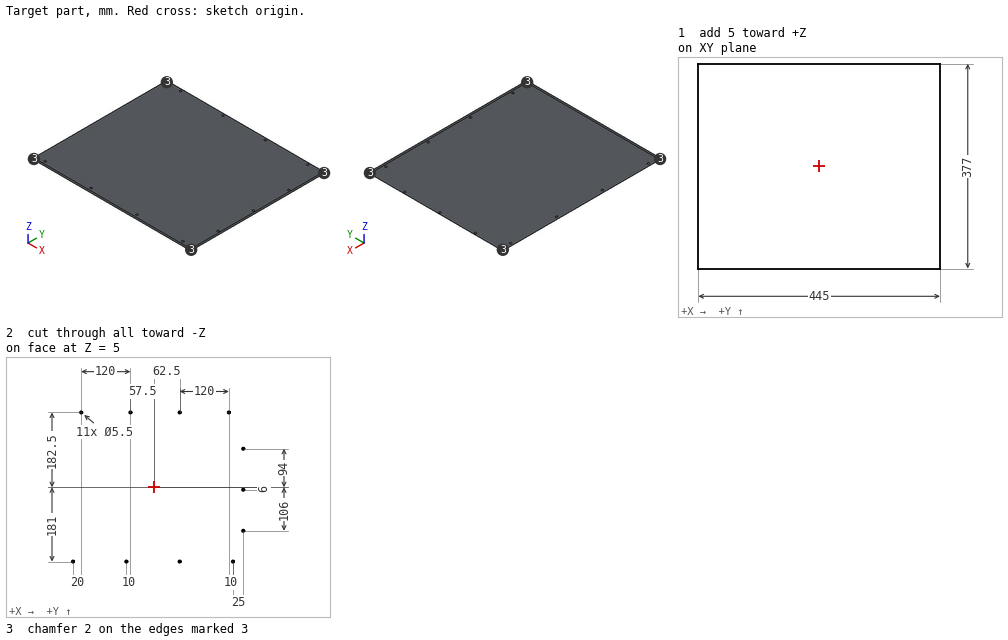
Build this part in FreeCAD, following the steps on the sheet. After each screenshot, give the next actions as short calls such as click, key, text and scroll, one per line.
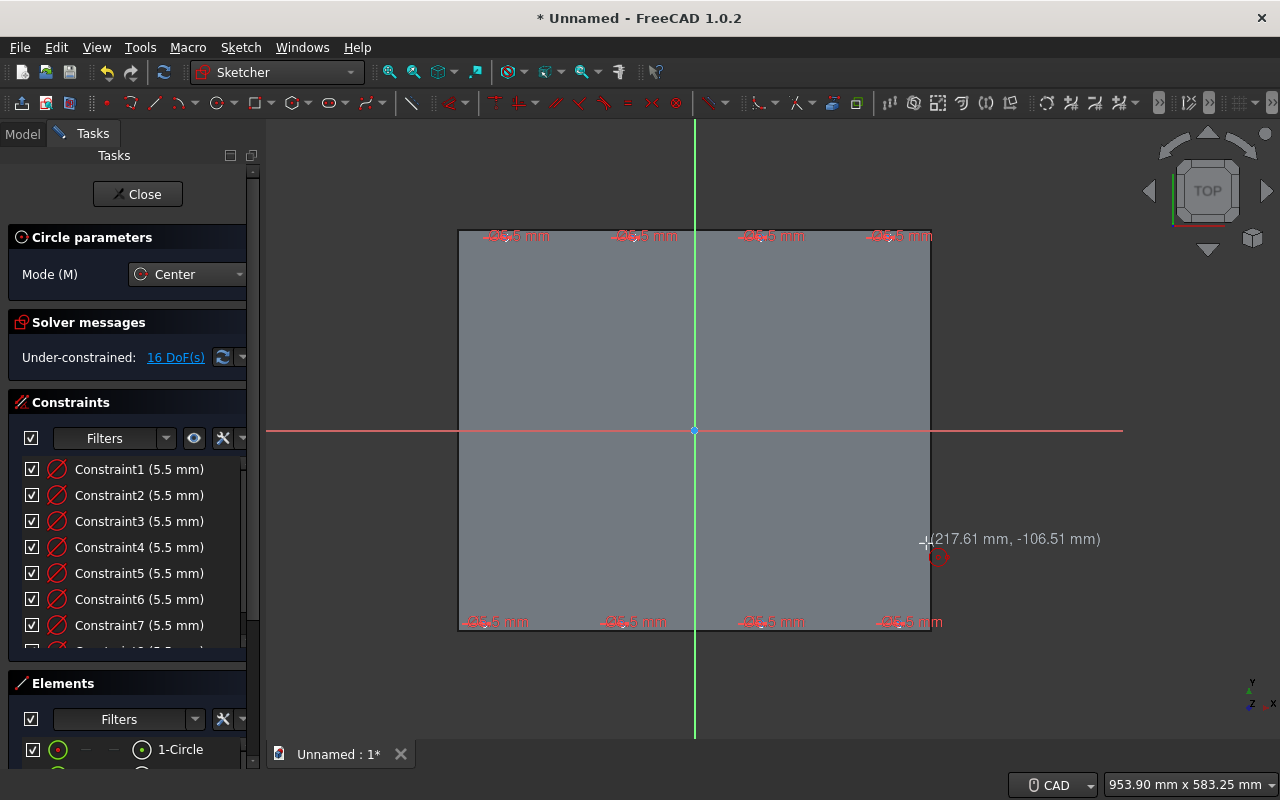
click(926, 543)
move(928, 541)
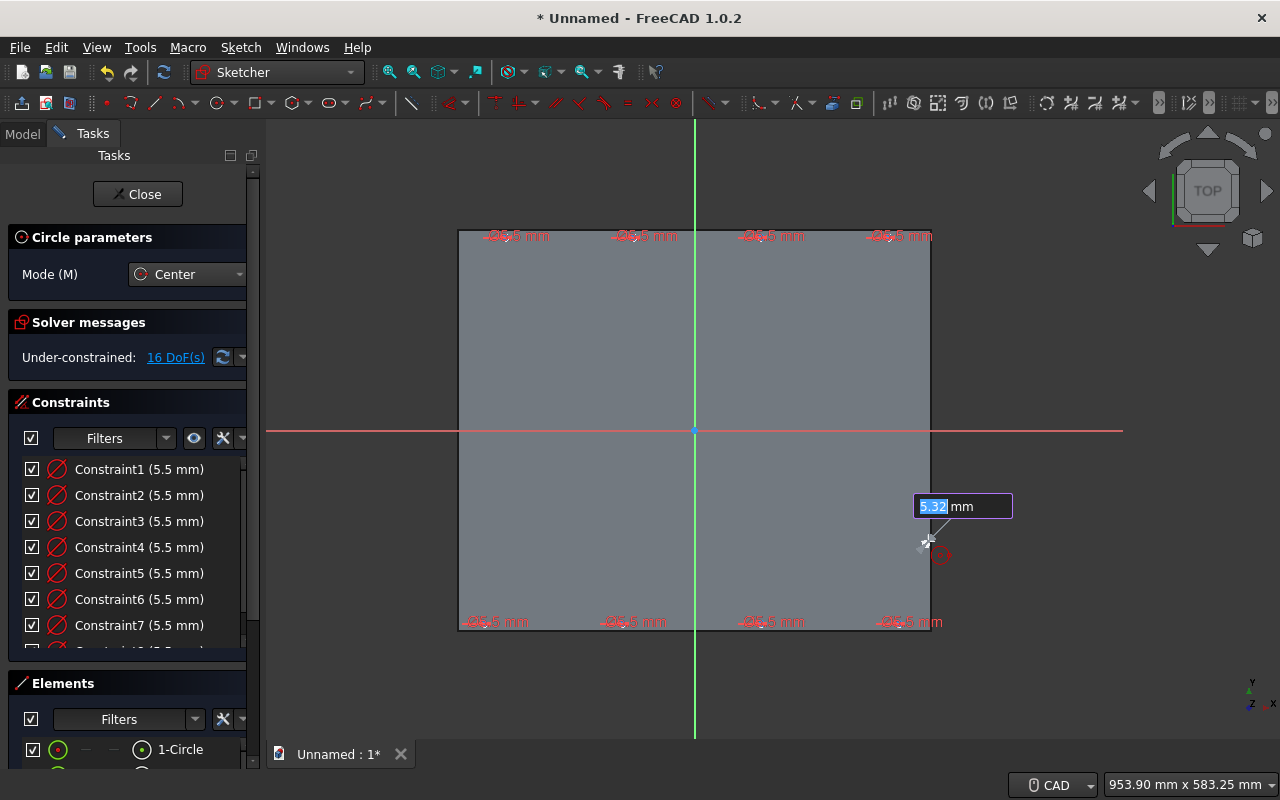
text(5.5)
key(Return)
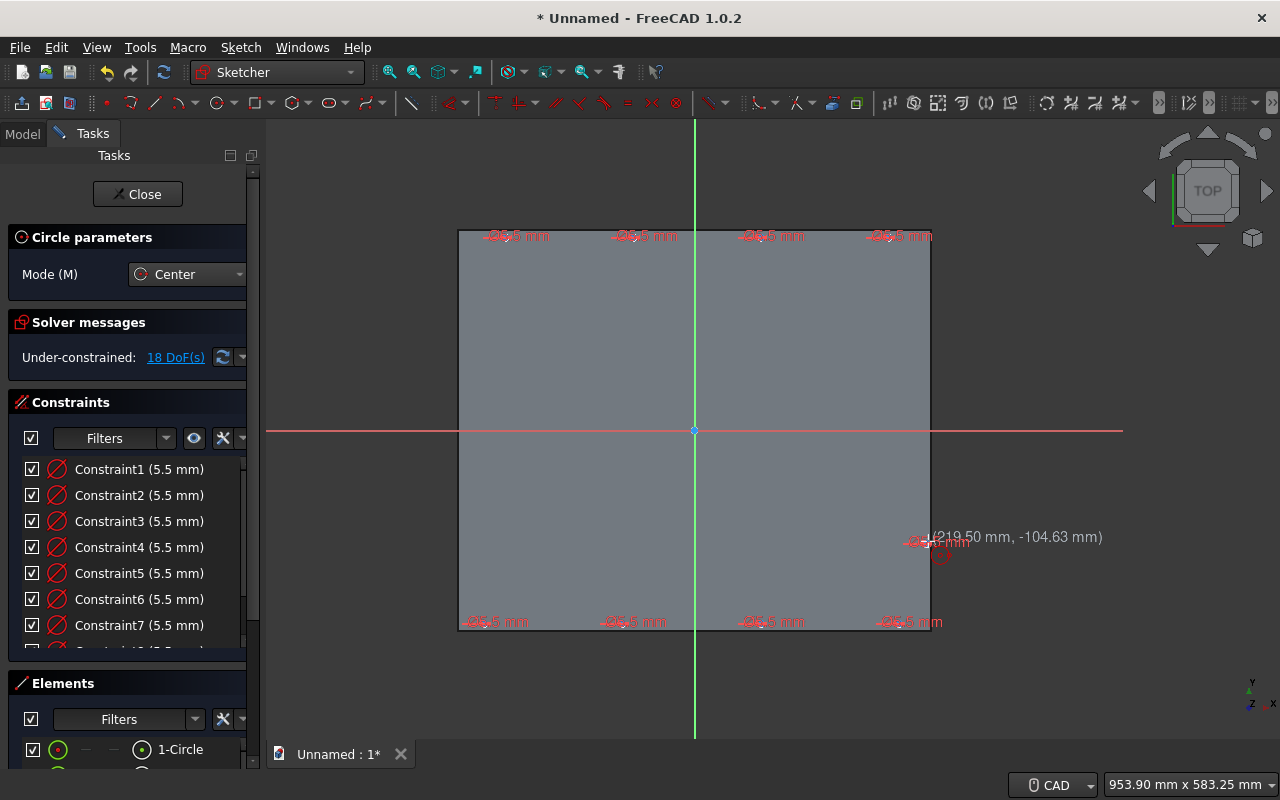
scroll(926, 437, up, 11)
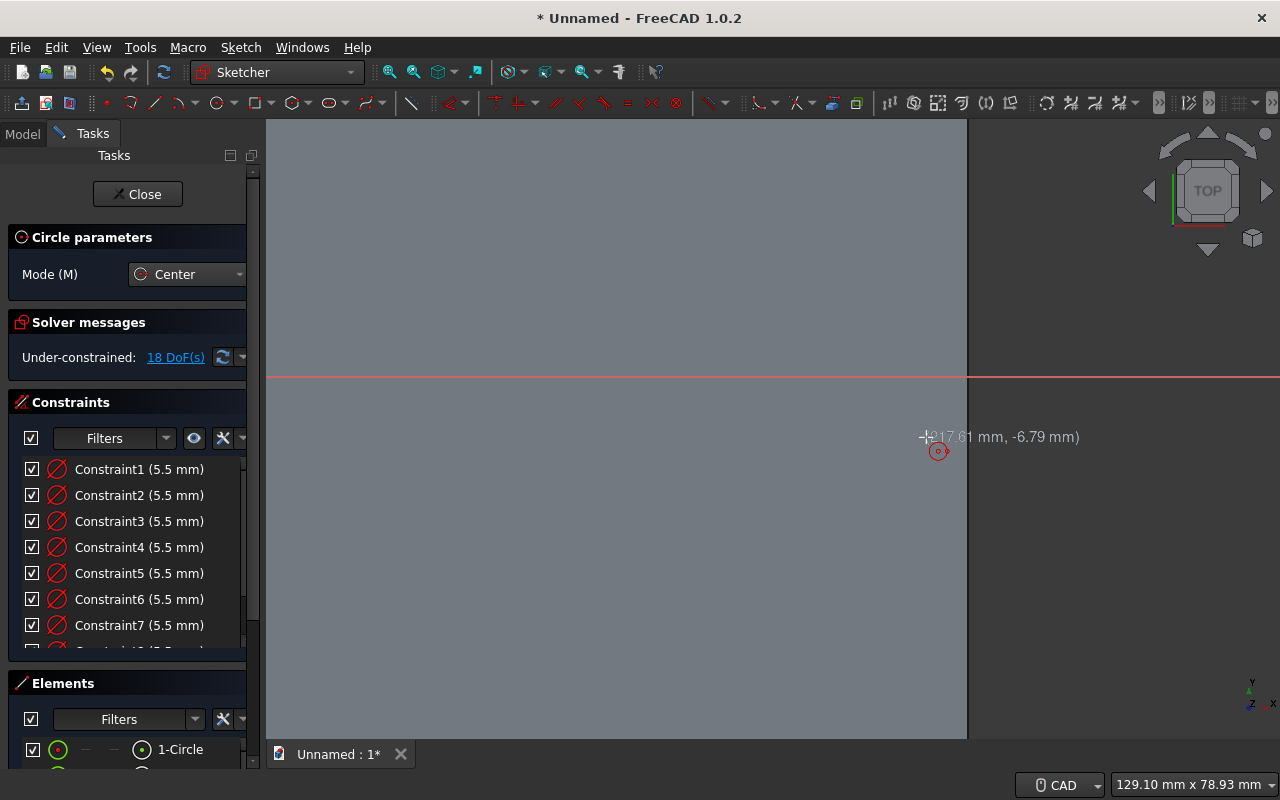
scroll(926, 436, down, 11)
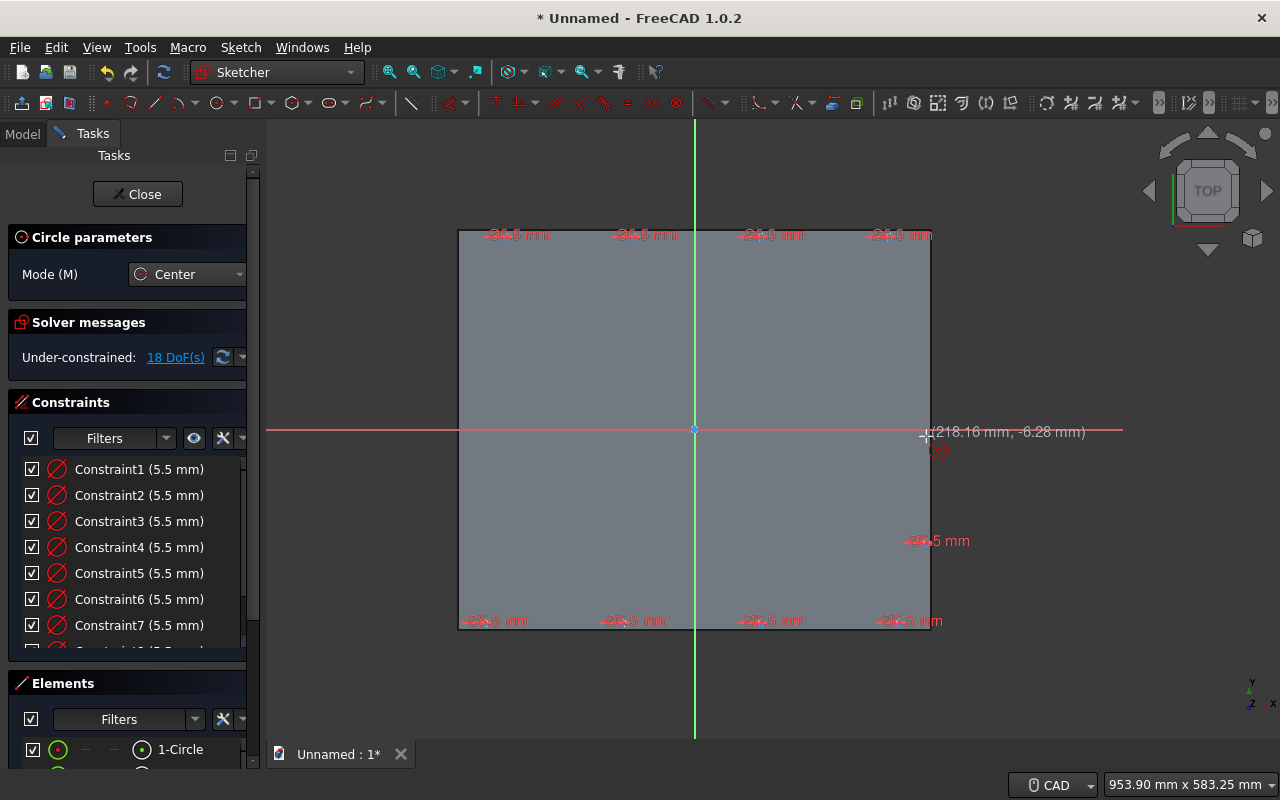
scroll(926, 436, up, 5)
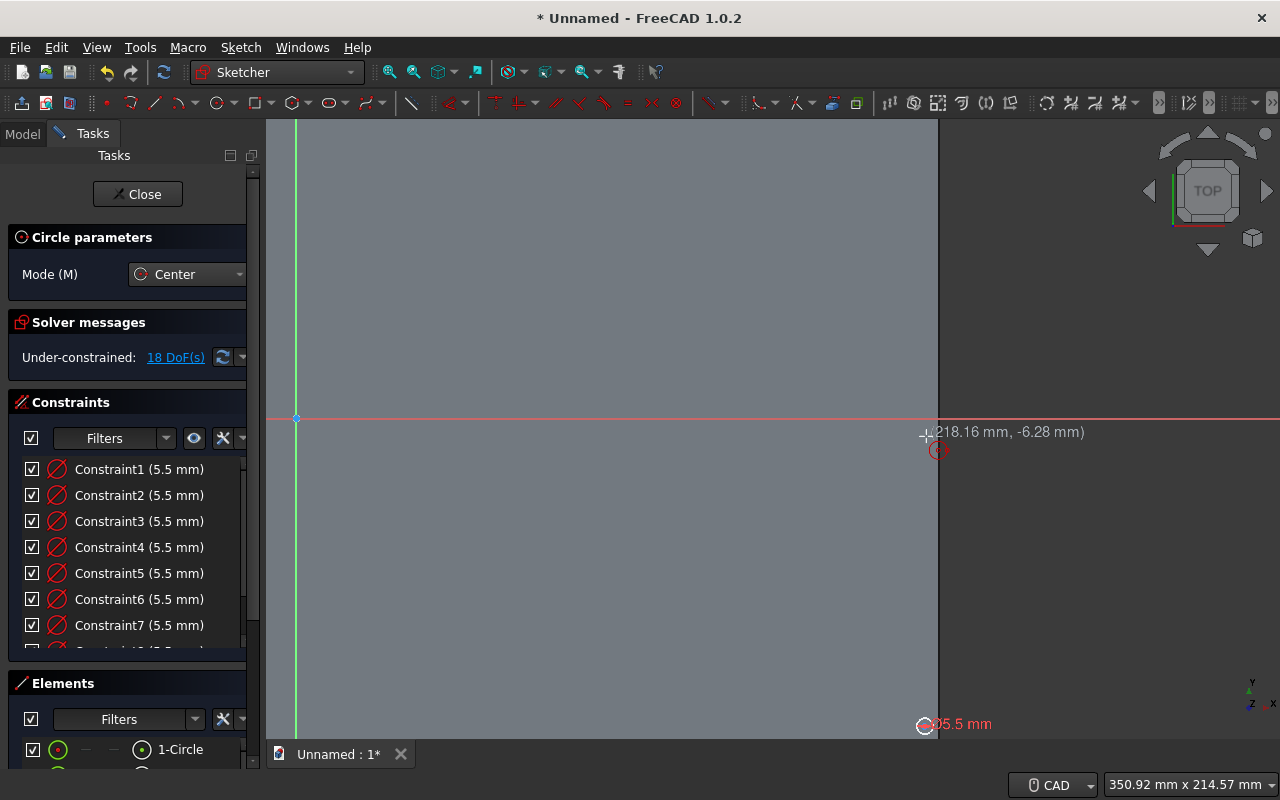
click(925, 436)
move(930, 441)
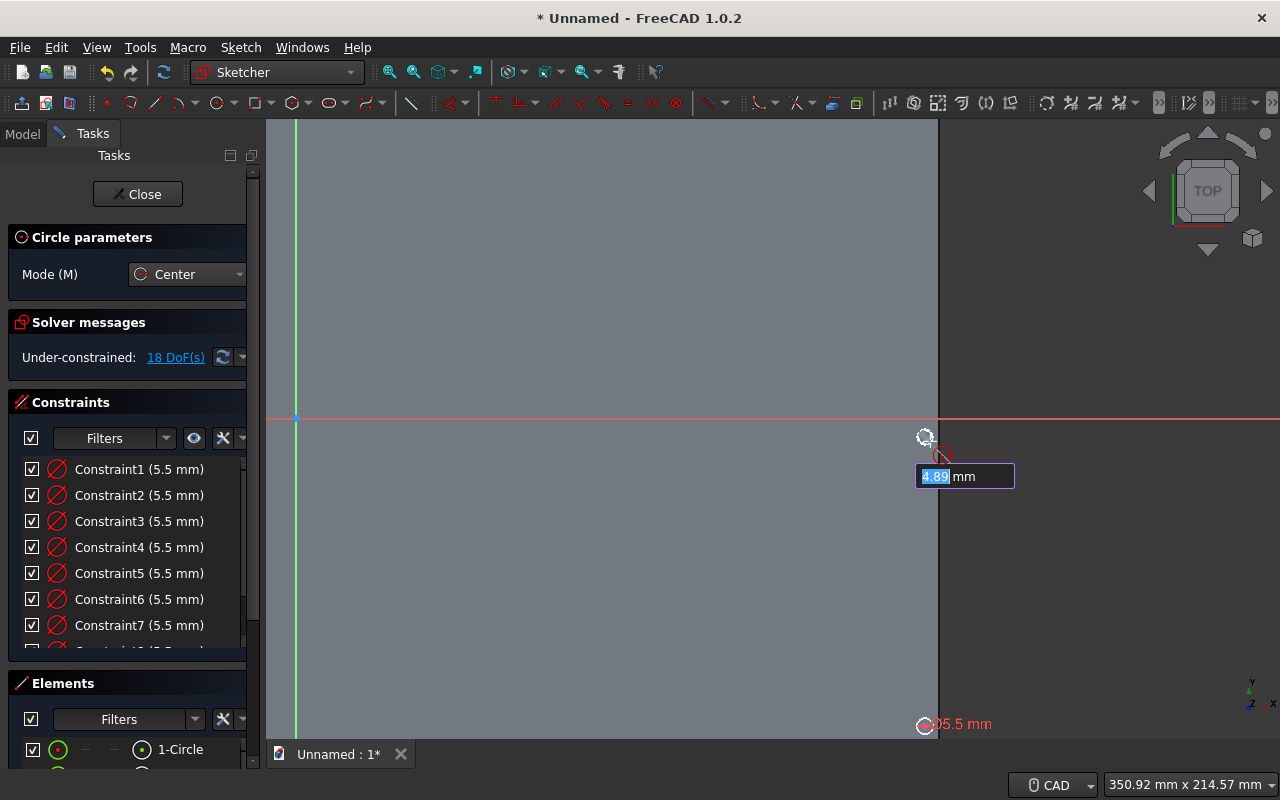
text(5.5)
key(Return)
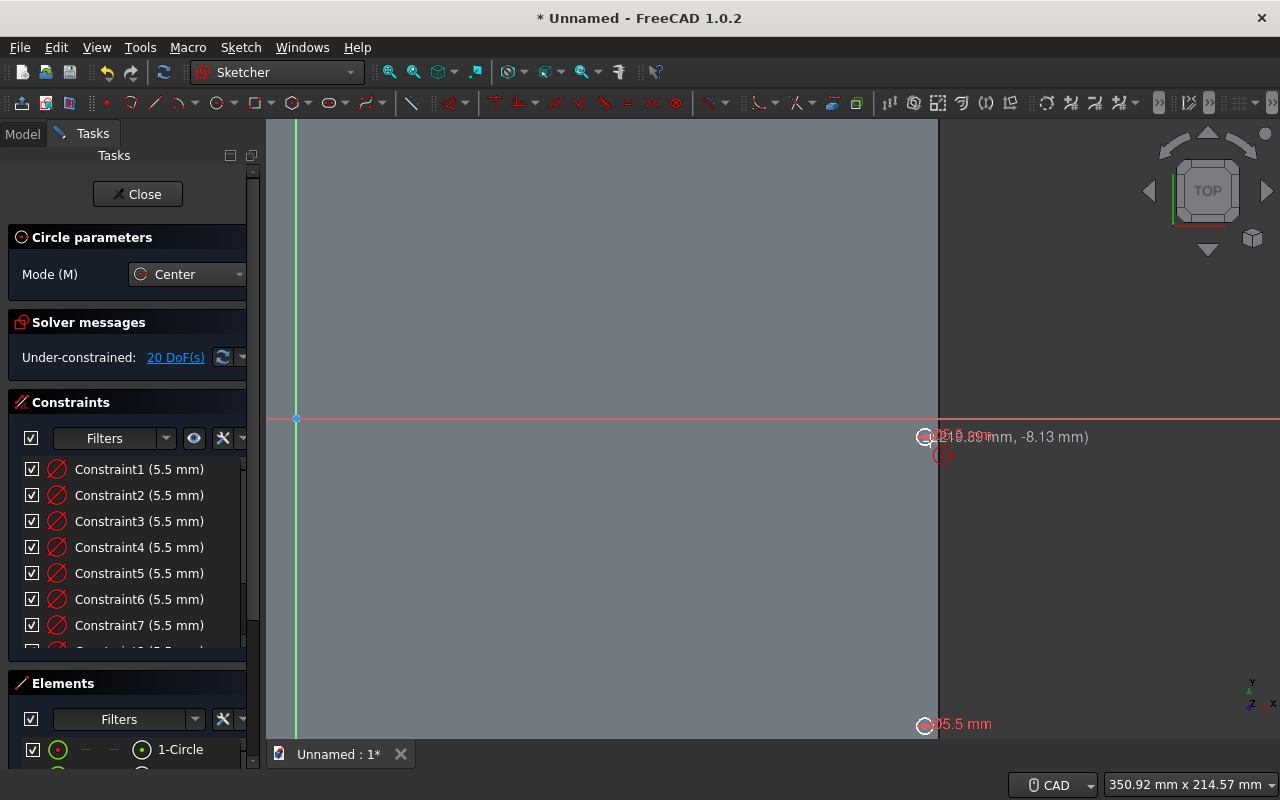
scroll(925, 436, down, 5)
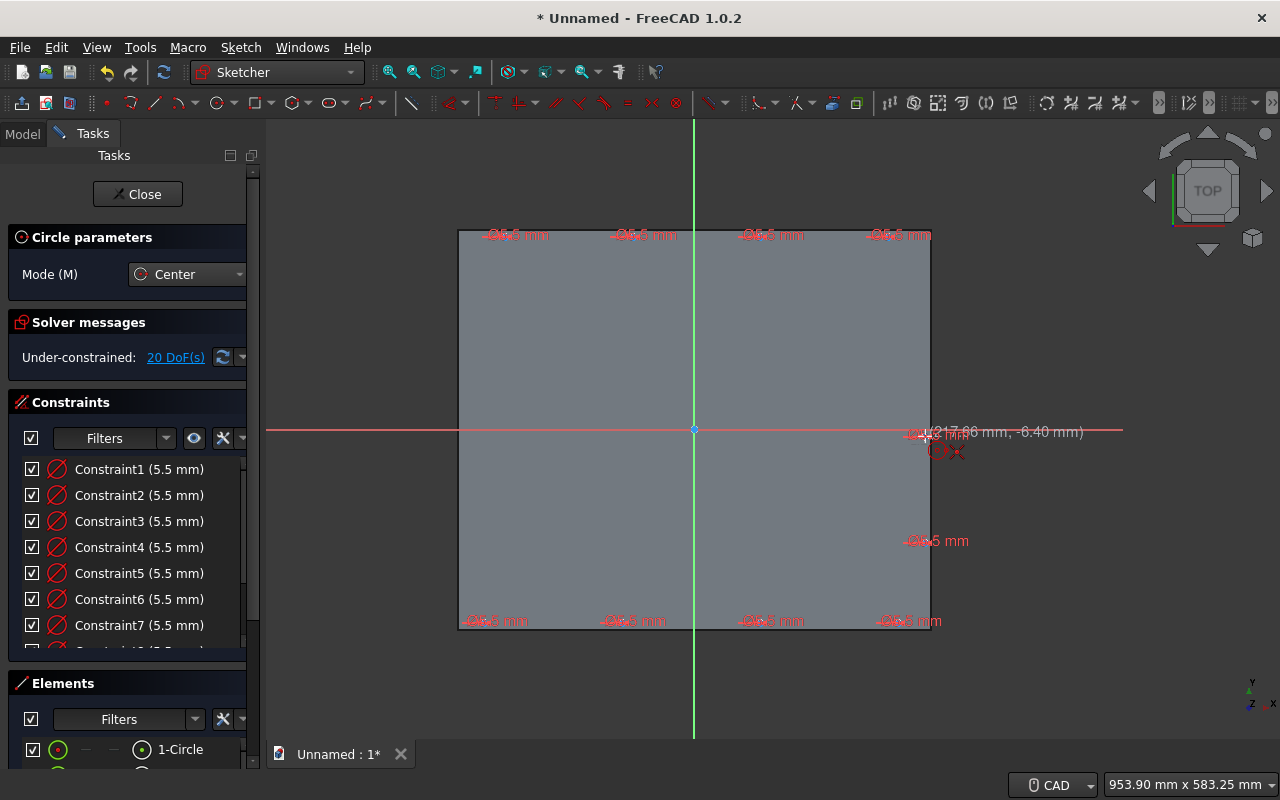
scroll(925, 330, up, 11)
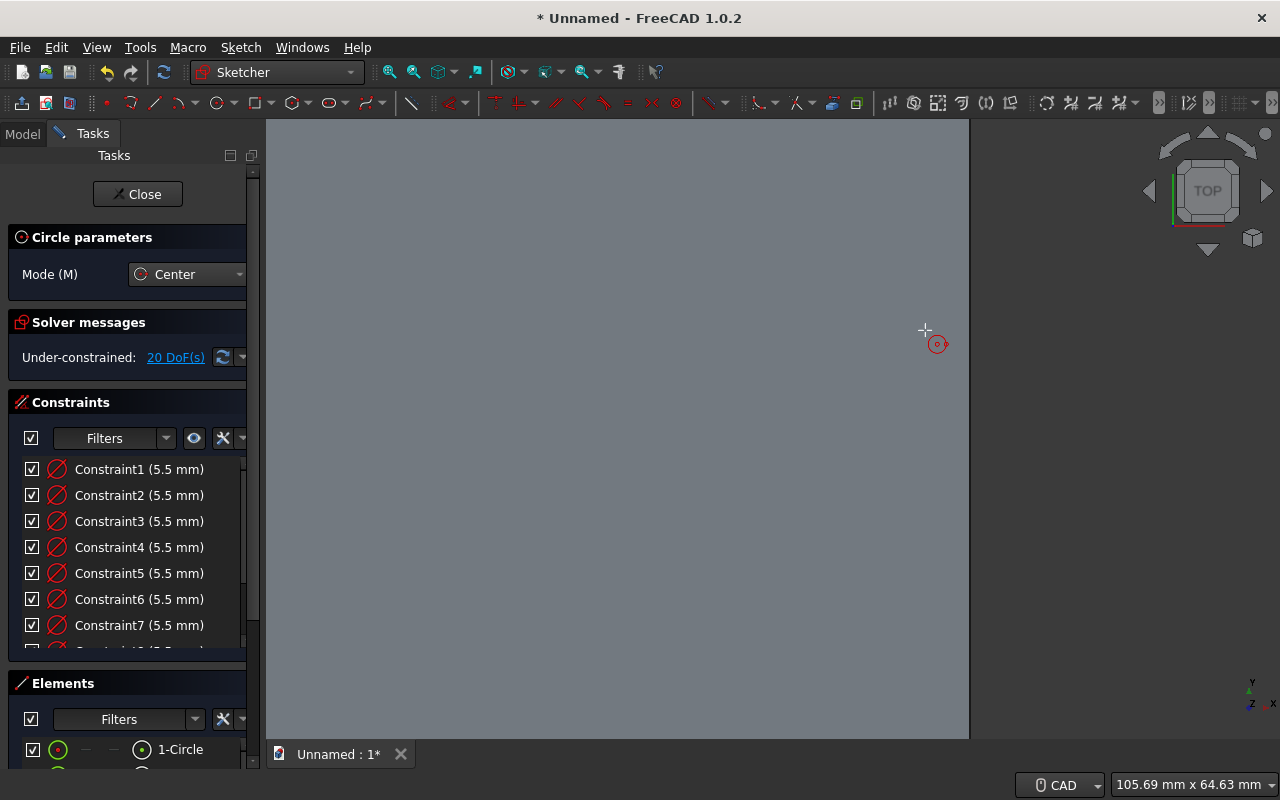
scroll(925, 330, down, 11)